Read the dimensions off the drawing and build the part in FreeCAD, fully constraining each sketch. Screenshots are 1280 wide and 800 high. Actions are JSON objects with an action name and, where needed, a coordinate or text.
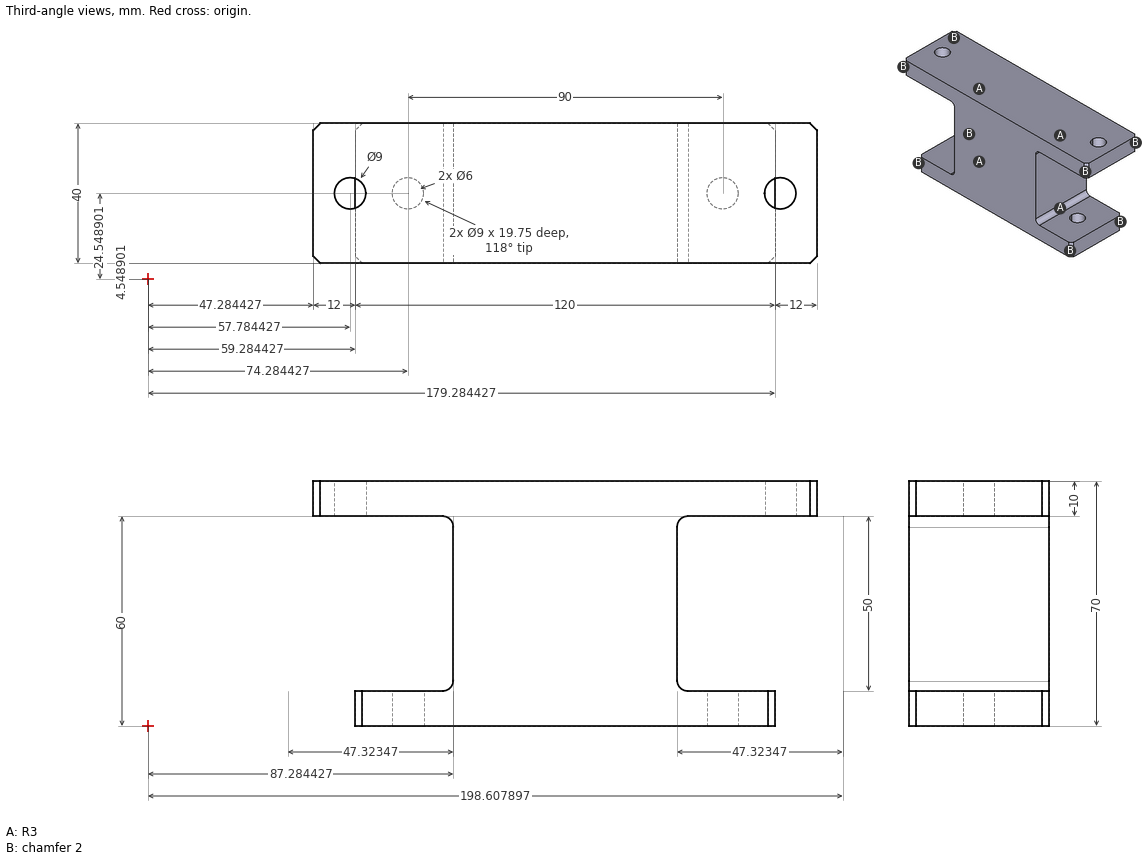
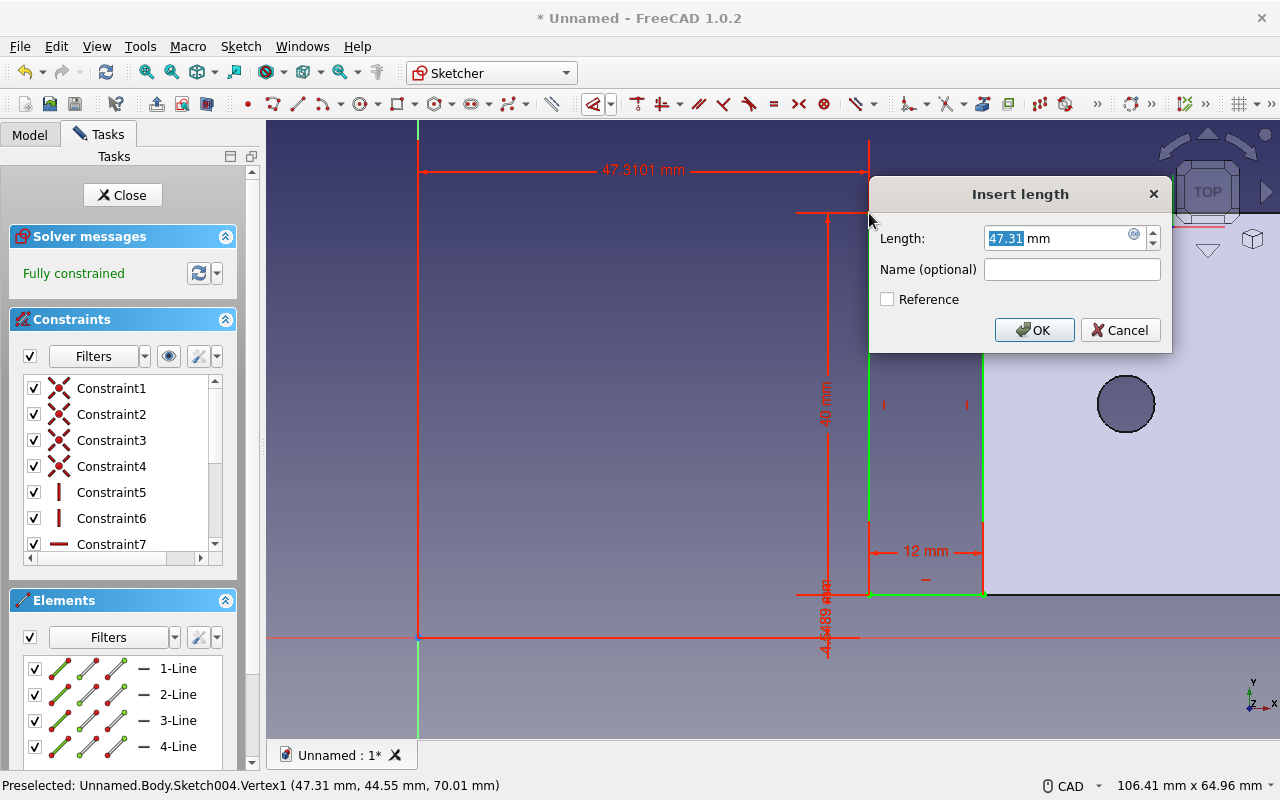
{"action": "type", "text": "47.284427"}
{"action": "key", "text": "Return"}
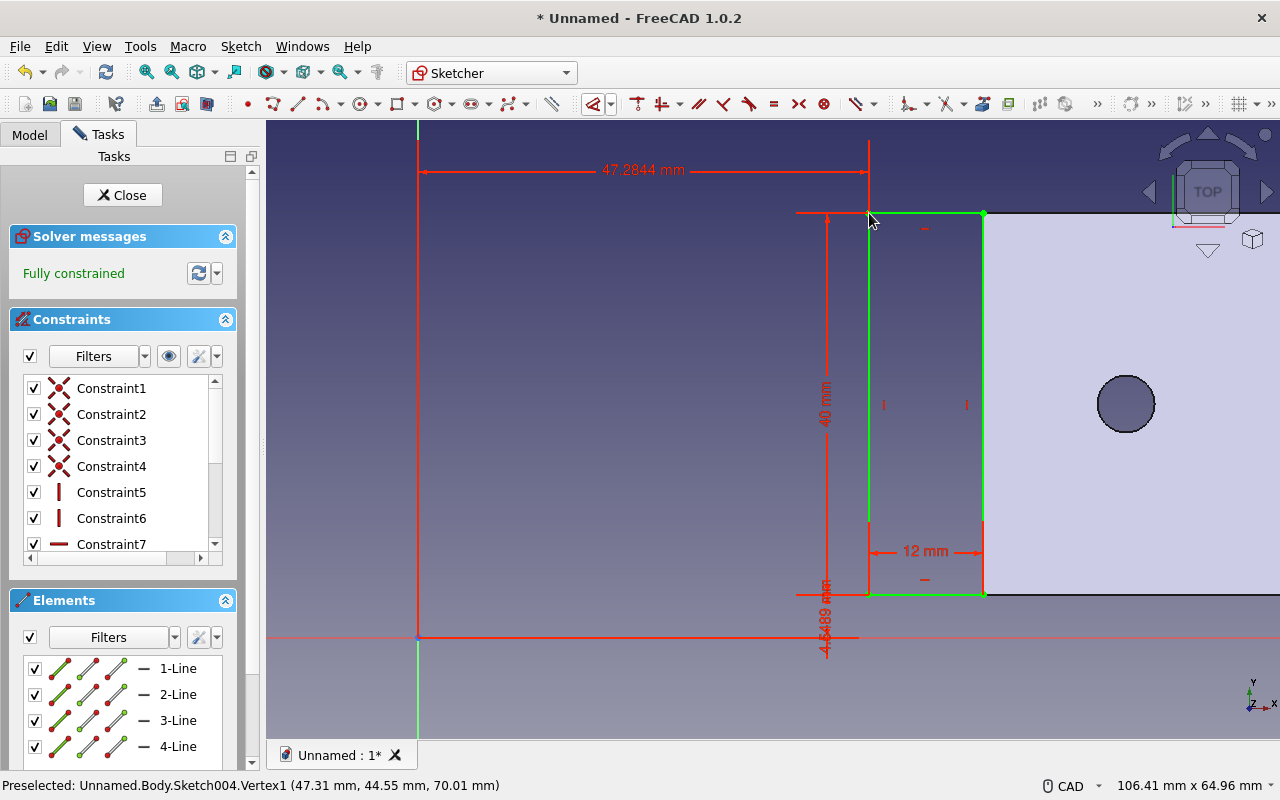
{"action": "left_click", "coordinate": [123, 195]}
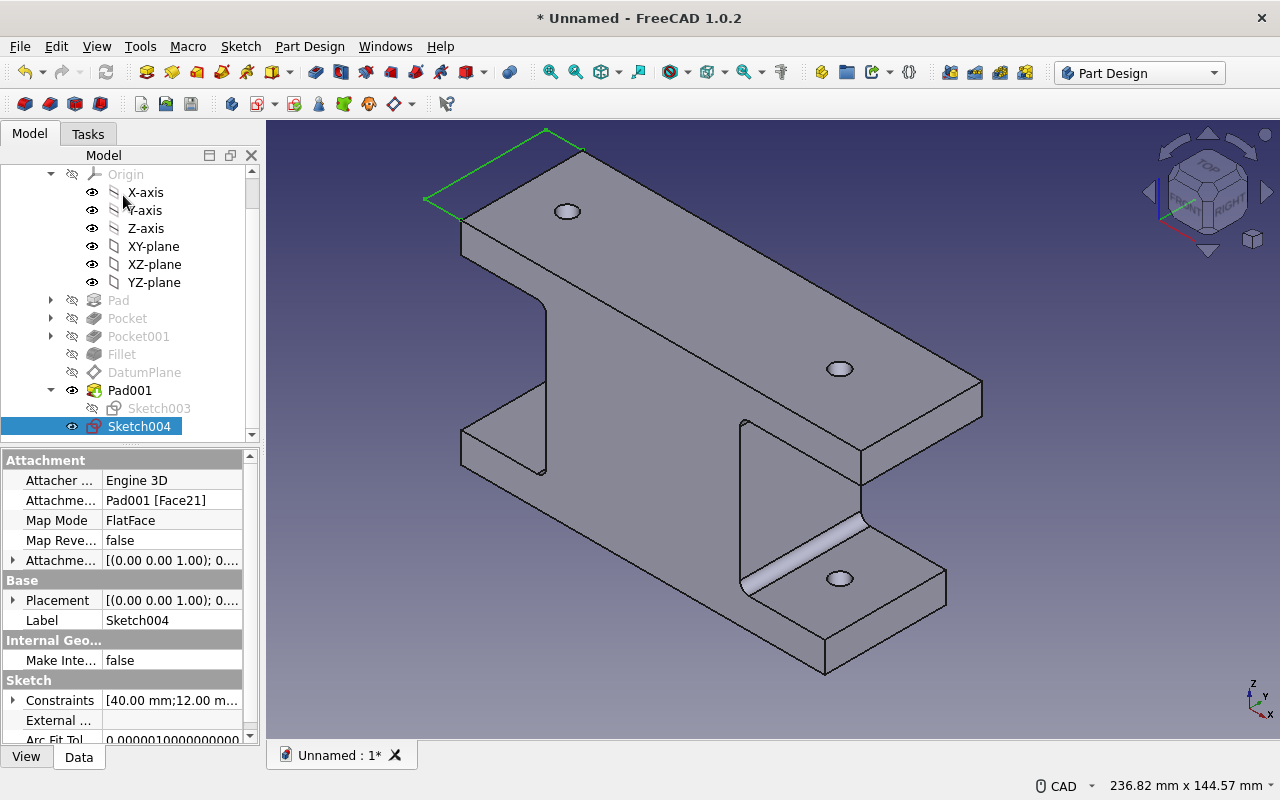
{"action": "left_click", "coordinate": [147, 72]}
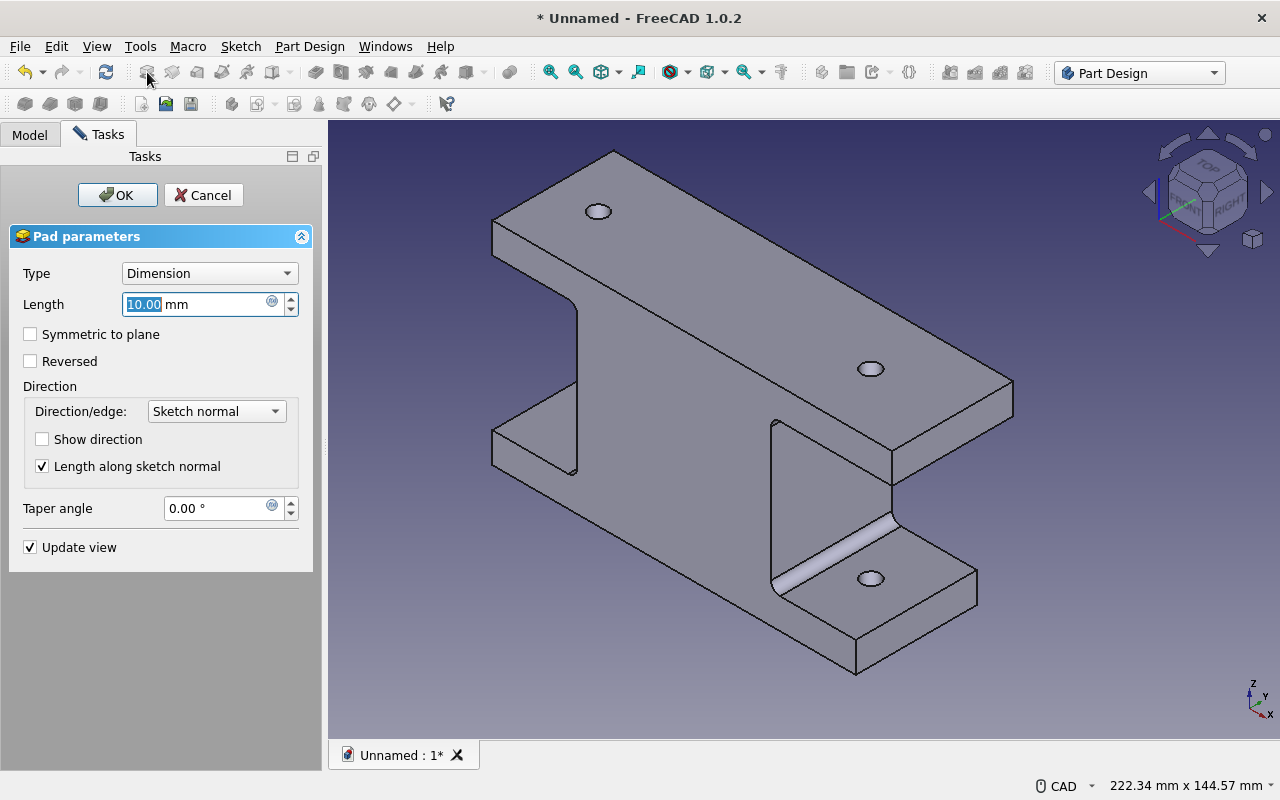
{"action": "type", "text": "10"}
{"action": "key", "text": "Tab"}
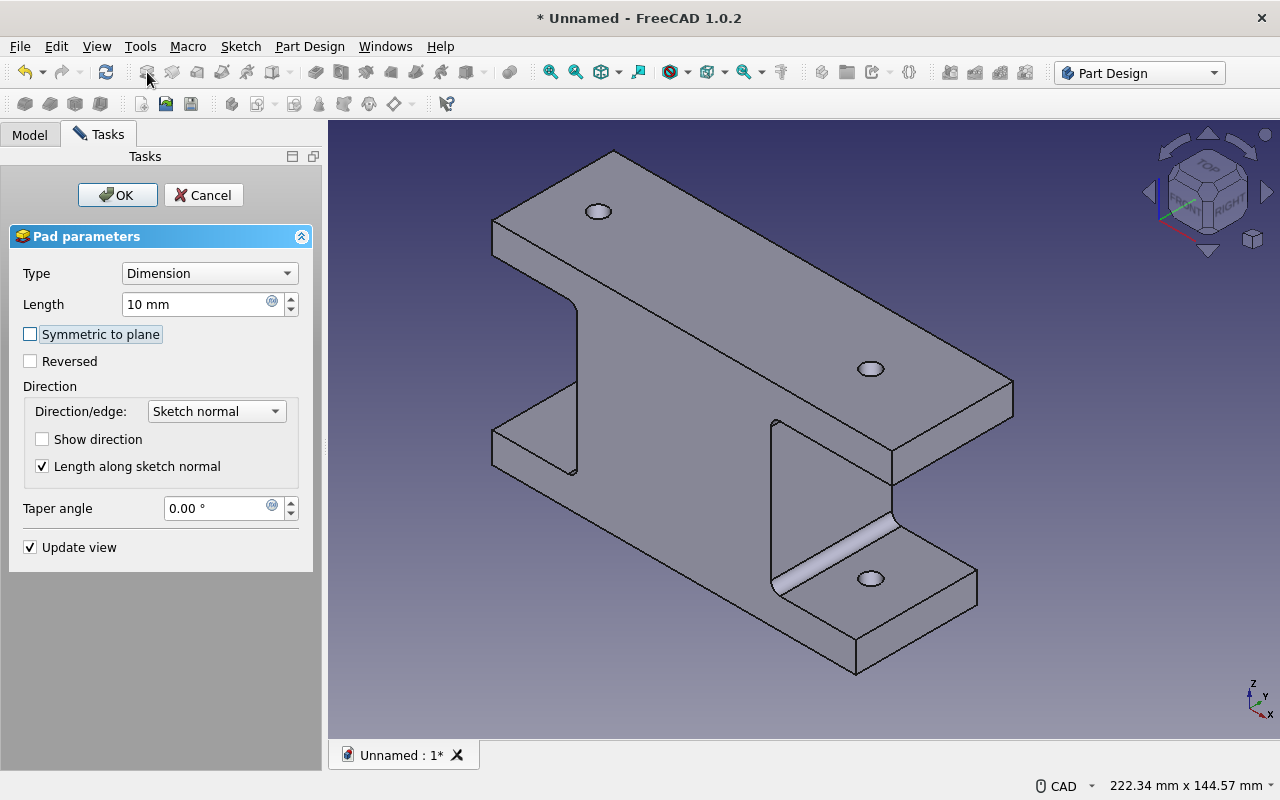
{"action": "left_click", "coordinate": [31, 361]}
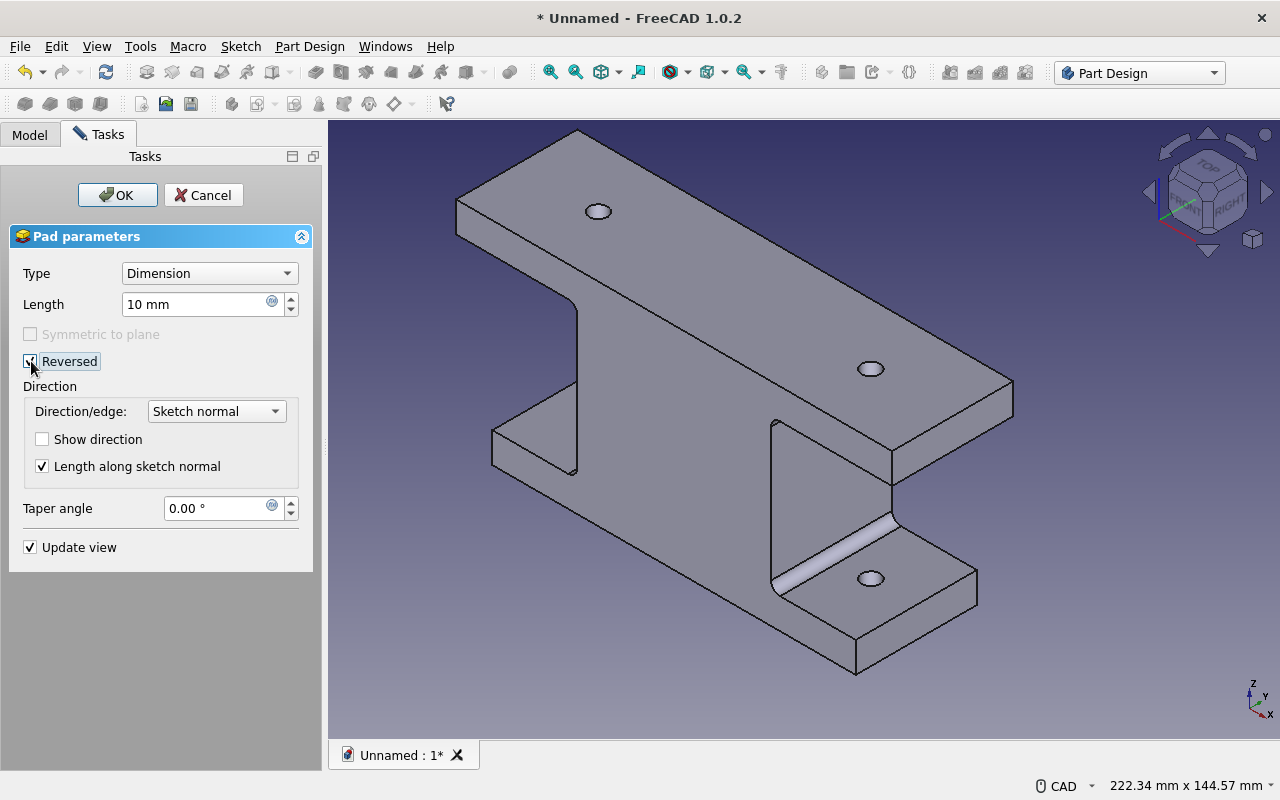
{"action": "left_click", "coordinate": [118, 195]}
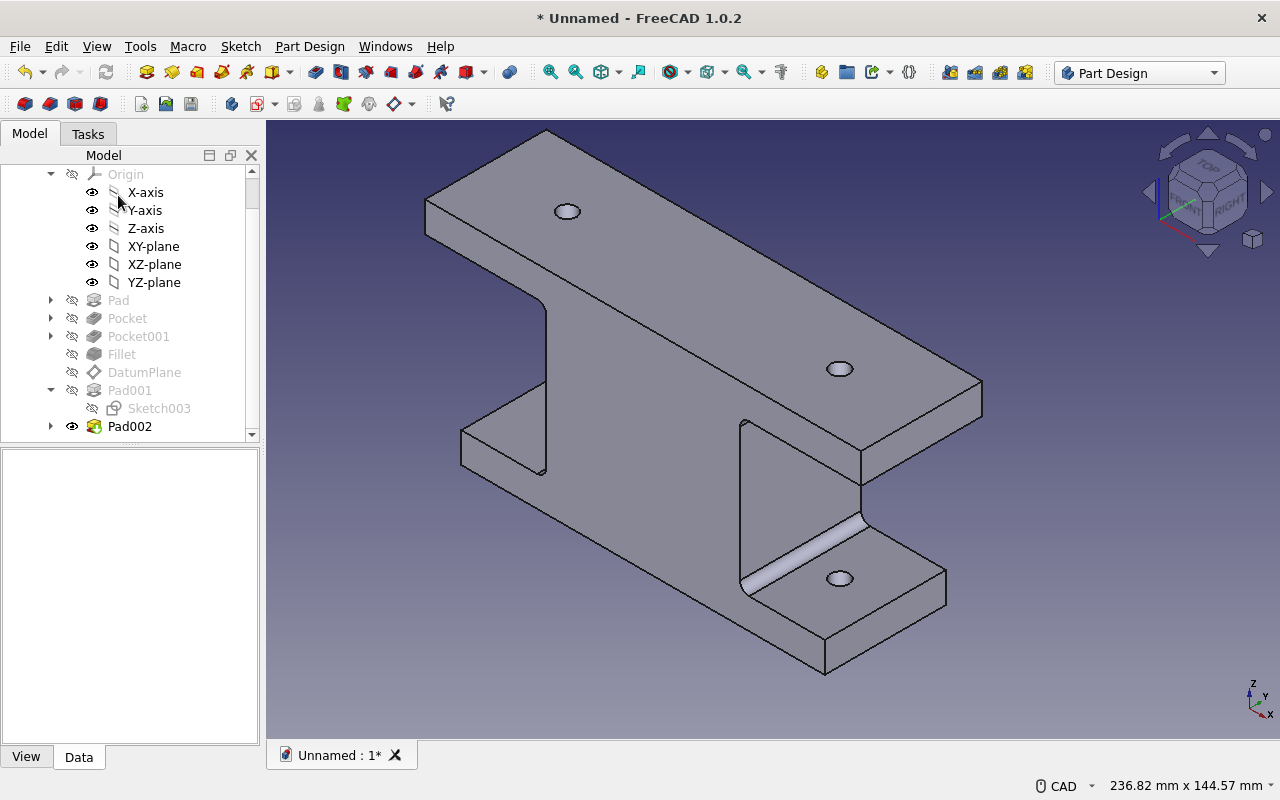
{"action": "left_click", "coordinate": [766, 325]}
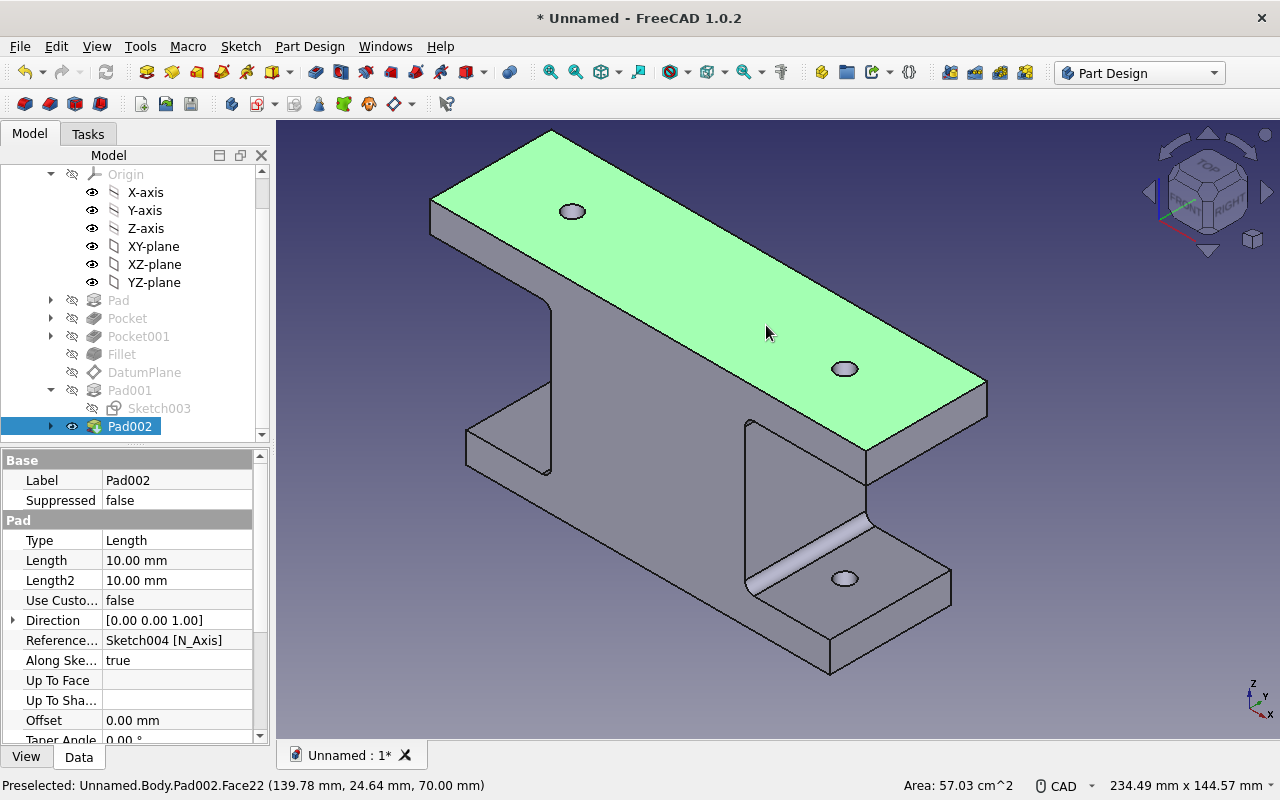
{"action": "left_click", "coordinate": [256, 104]}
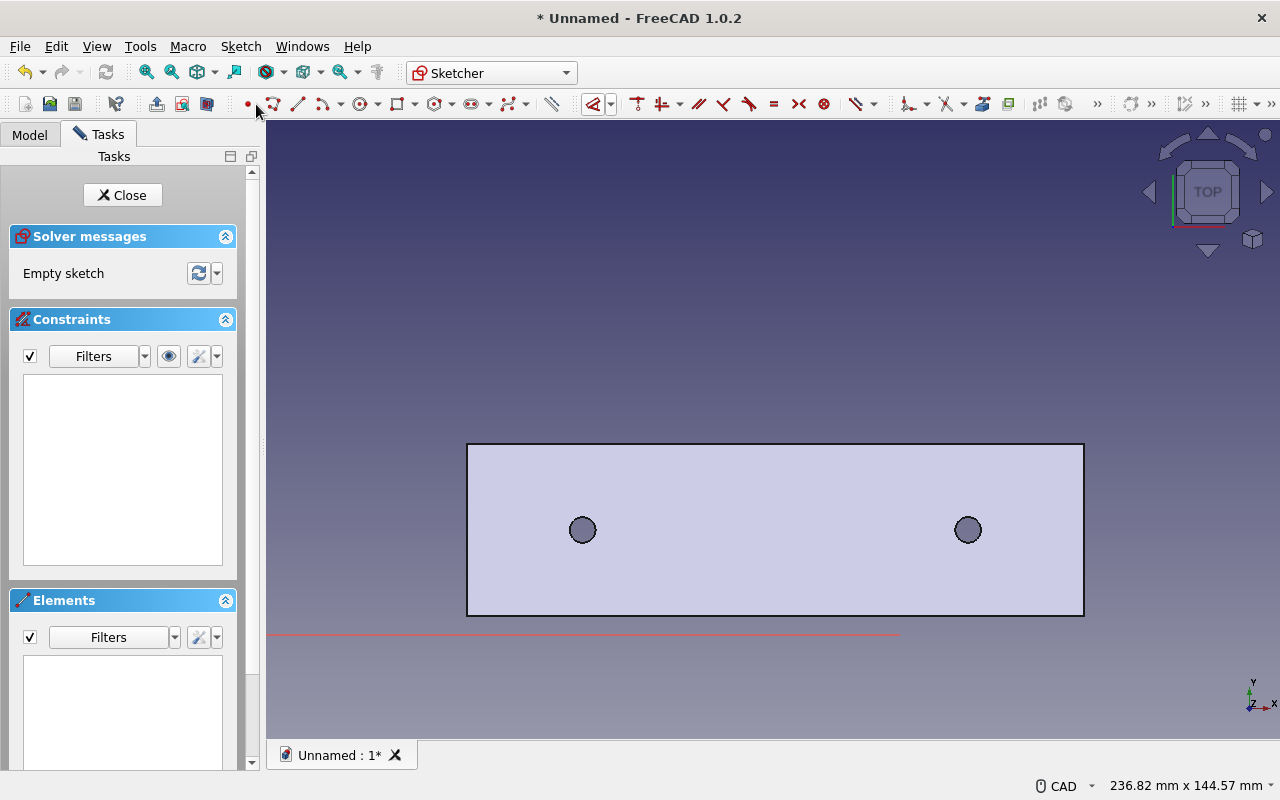
{"action": "scroll", "coordinate": [1074, 148], "scroll_direction": "down", "scroll_amount": 1}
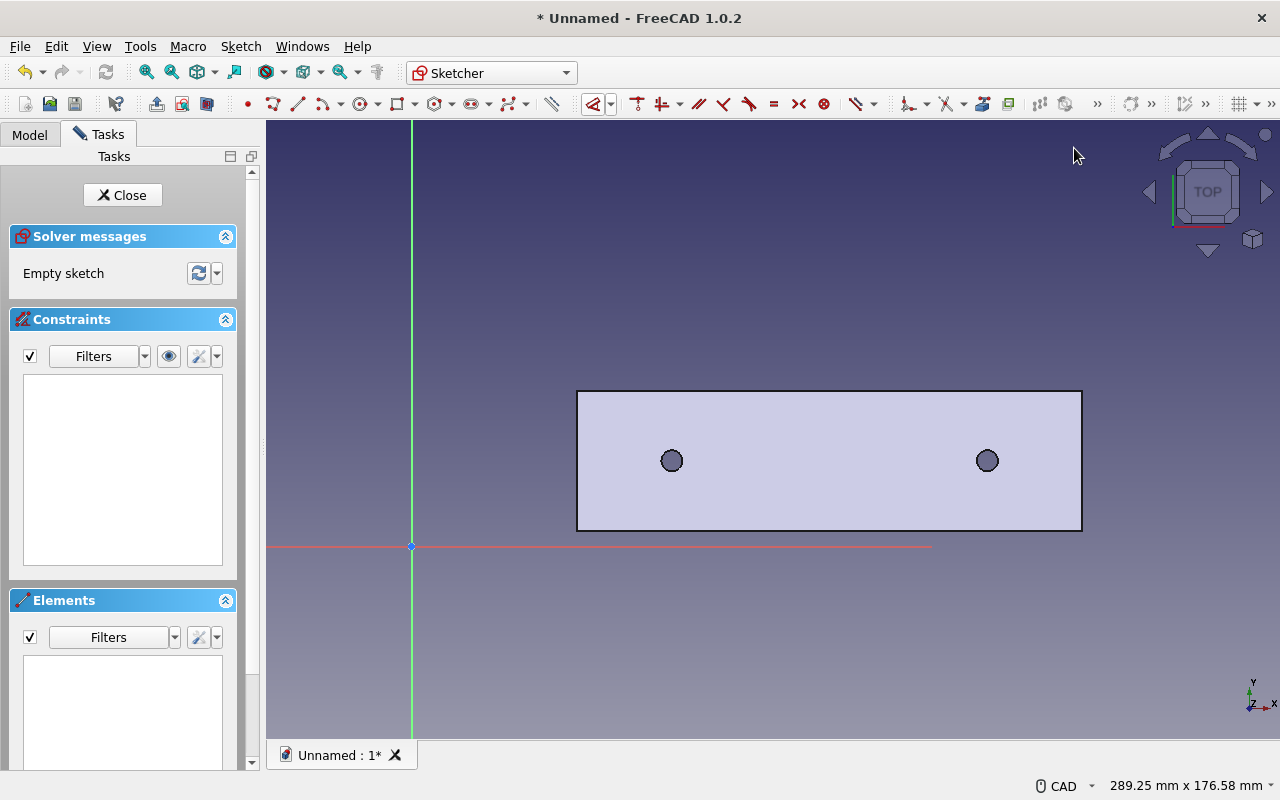
{"action": "key", "text": "g c"}